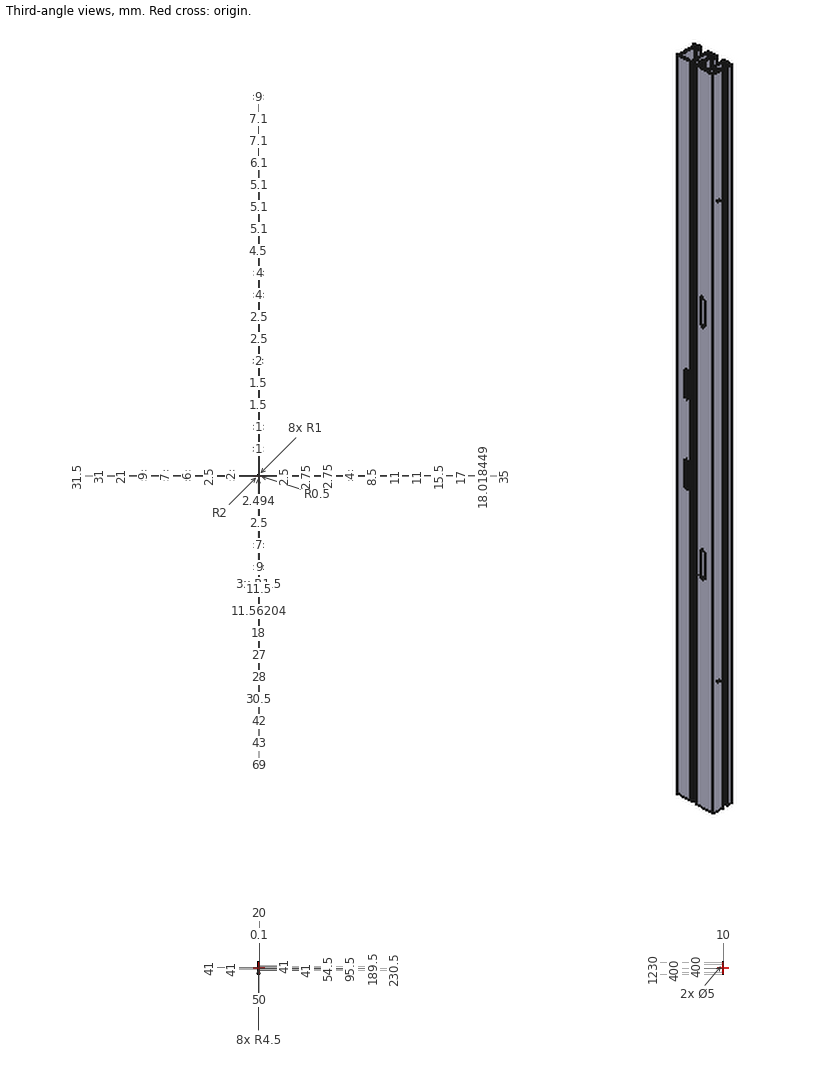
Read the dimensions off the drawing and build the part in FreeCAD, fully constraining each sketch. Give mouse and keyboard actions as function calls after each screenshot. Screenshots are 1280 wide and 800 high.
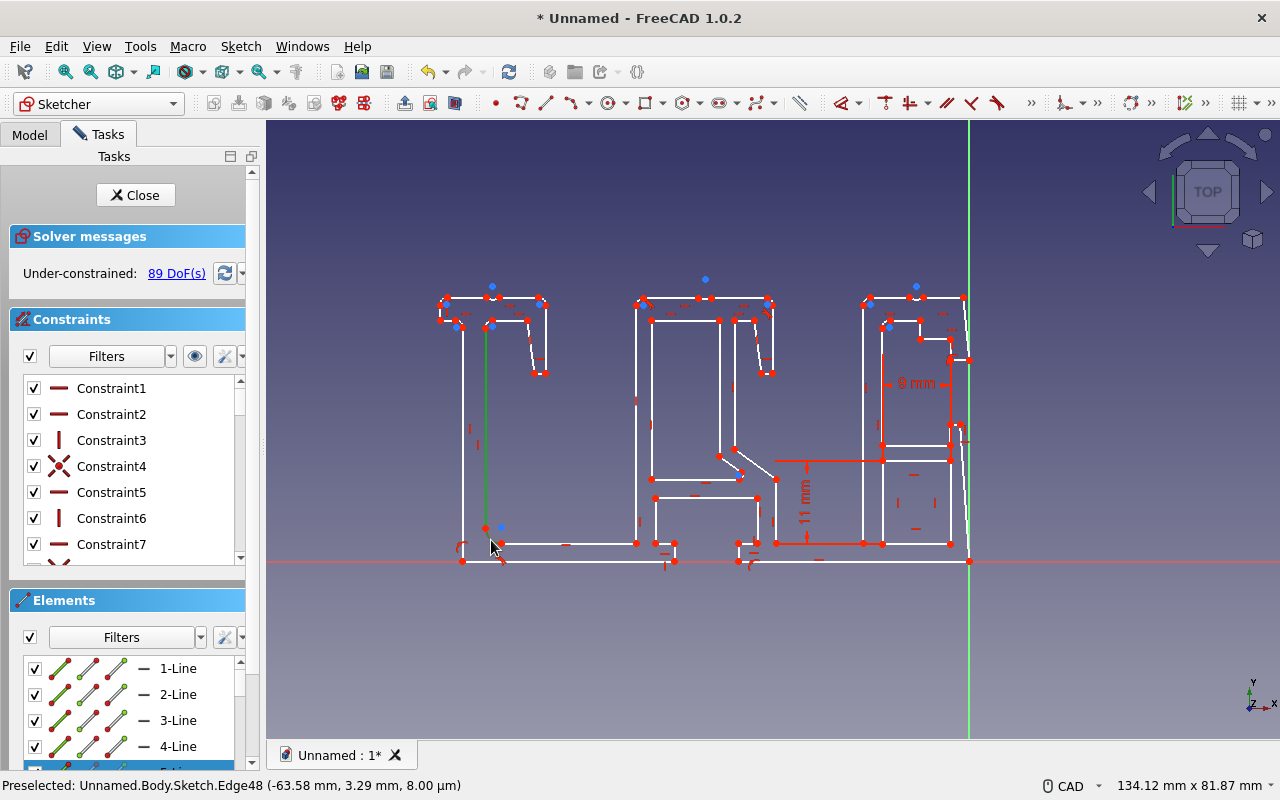
click(997, 104)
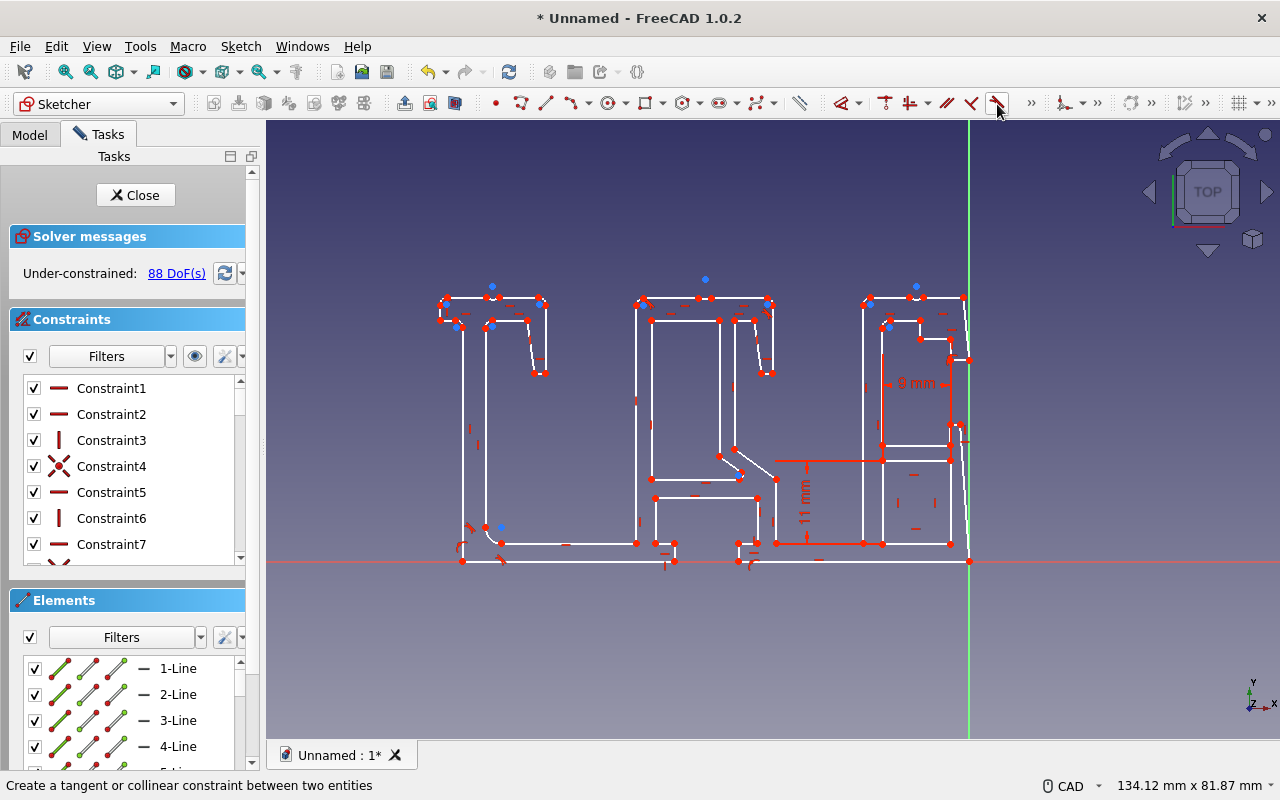
click(486, 468)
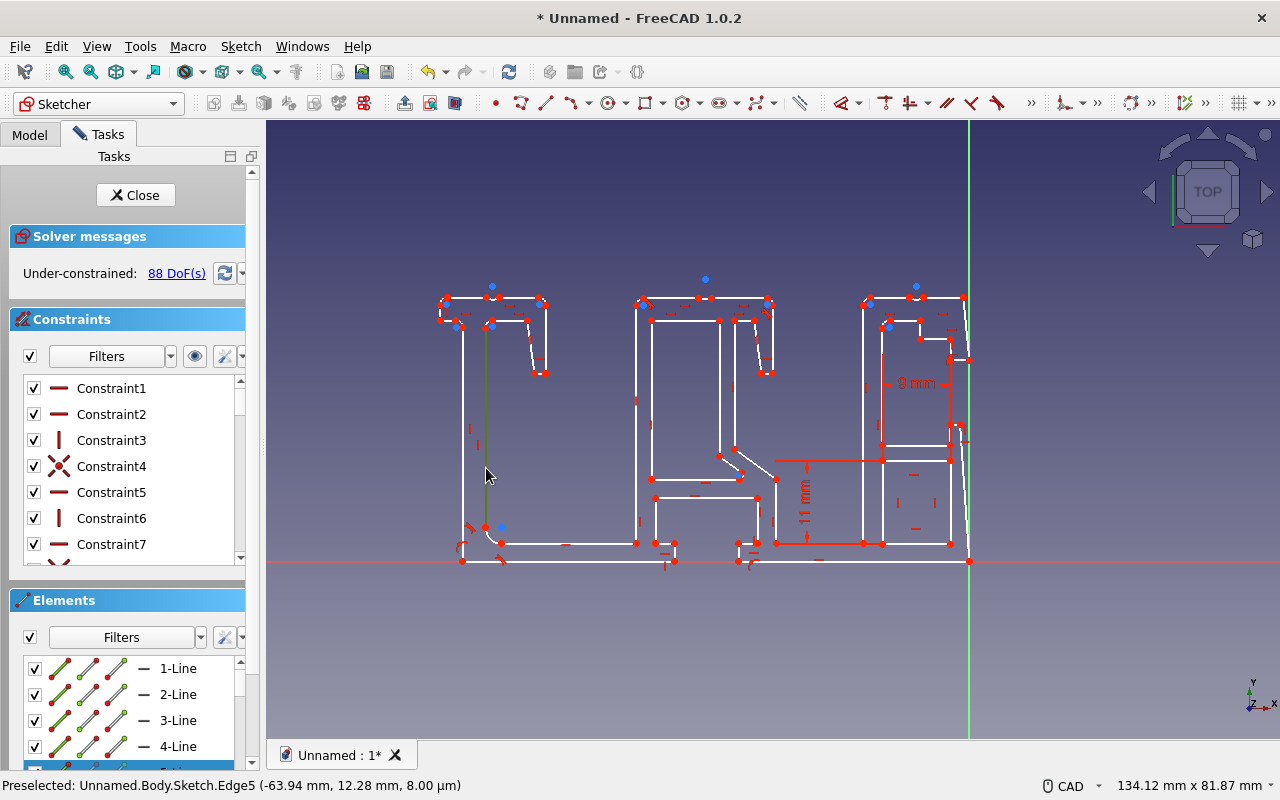
scroll(487, 323, up, 5)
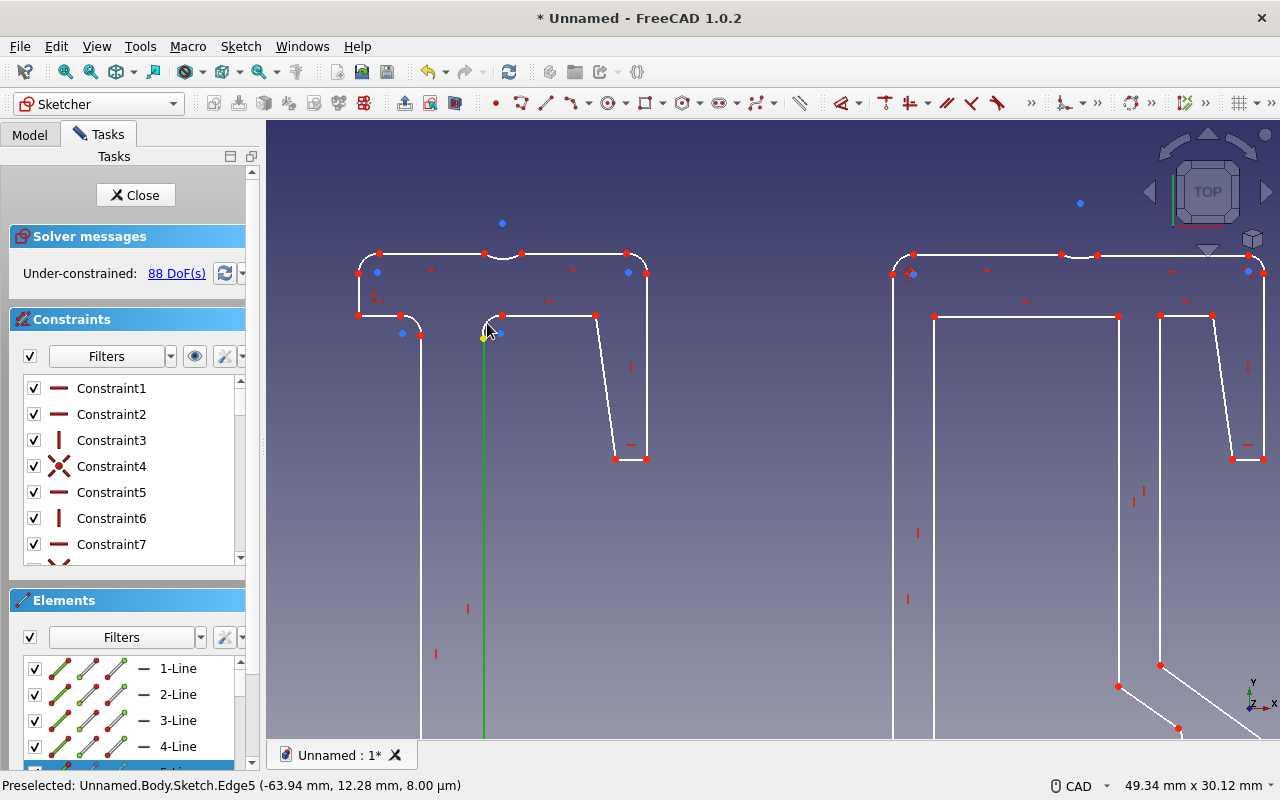
click(487, 322)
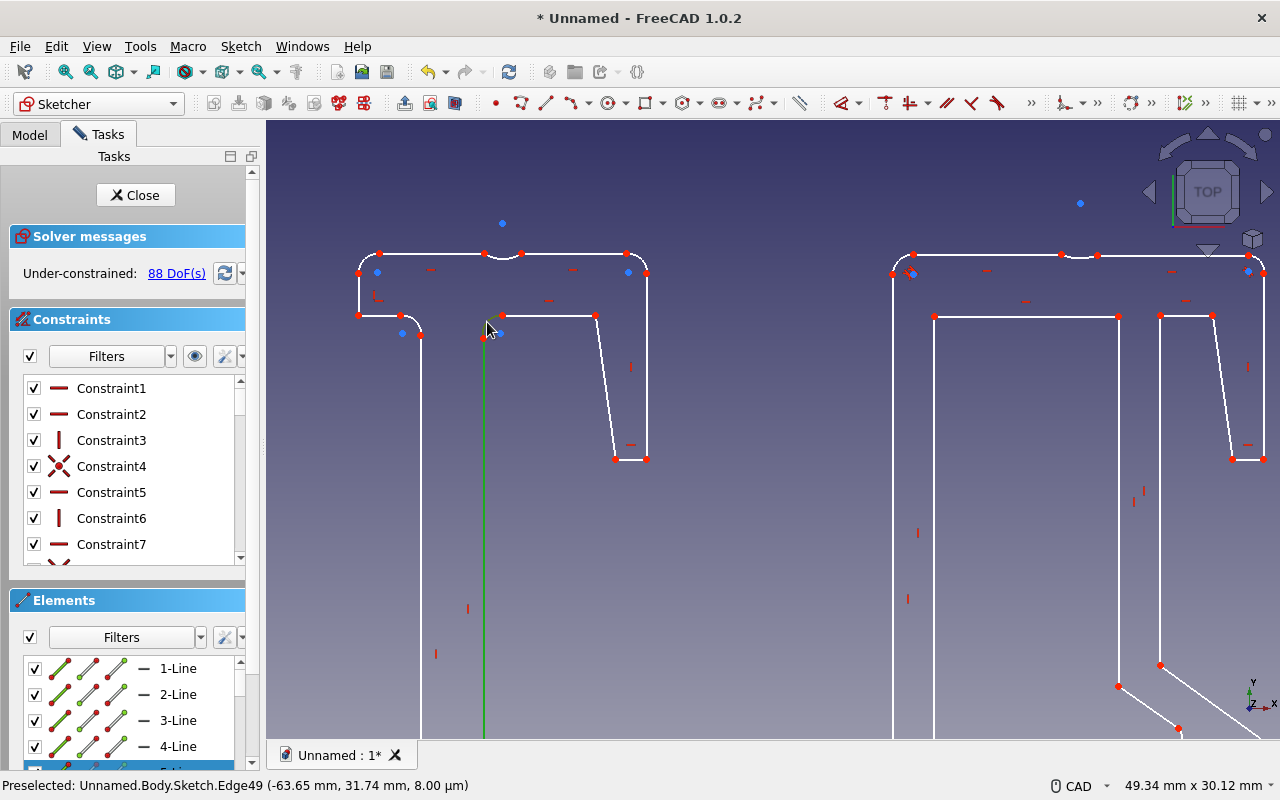
click(997, 104)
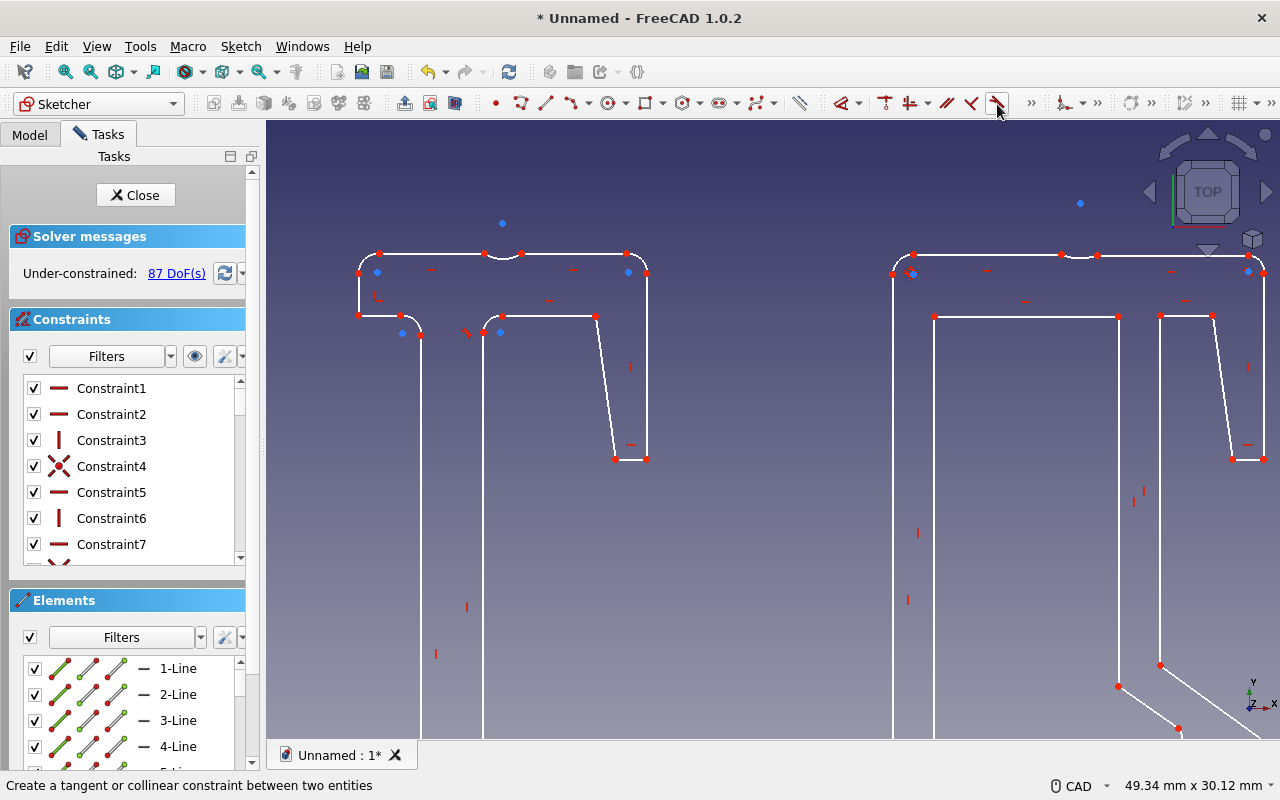
click(531, 316)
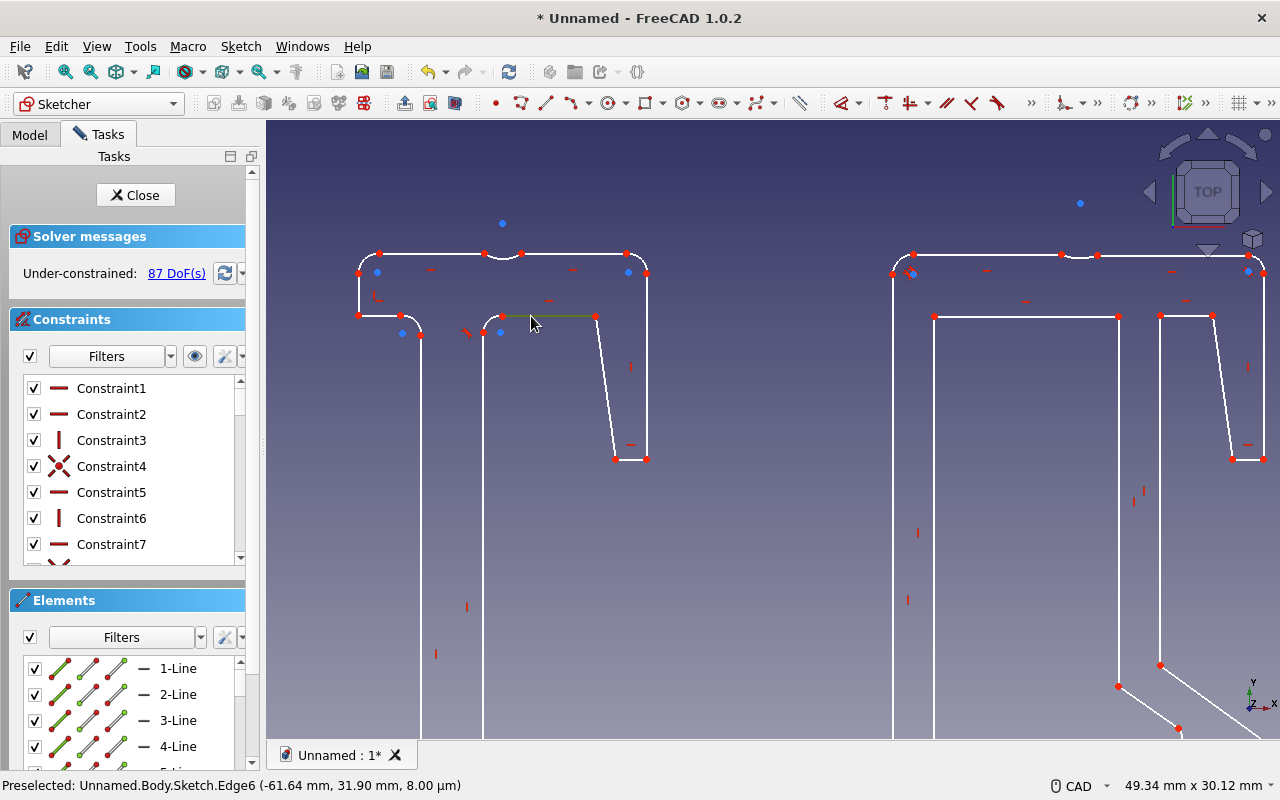
click(489, 320)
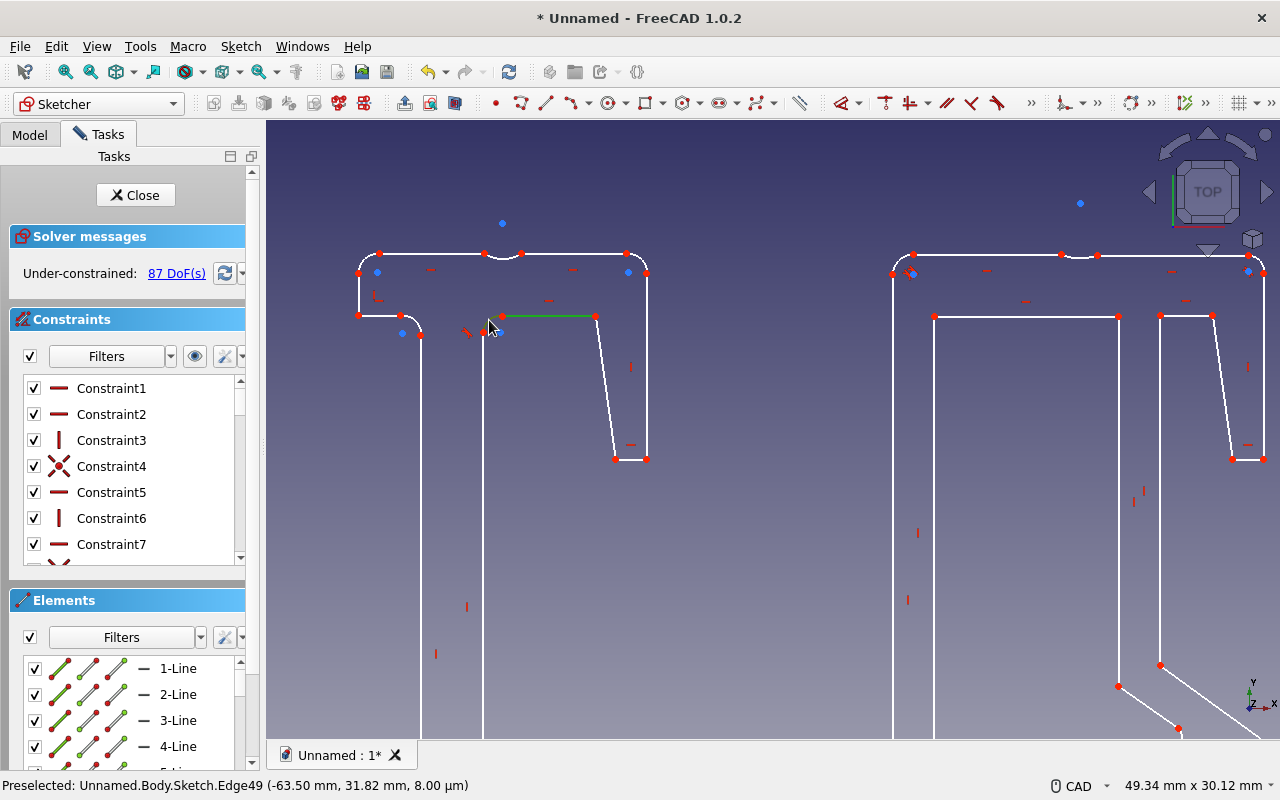
click(997, 104)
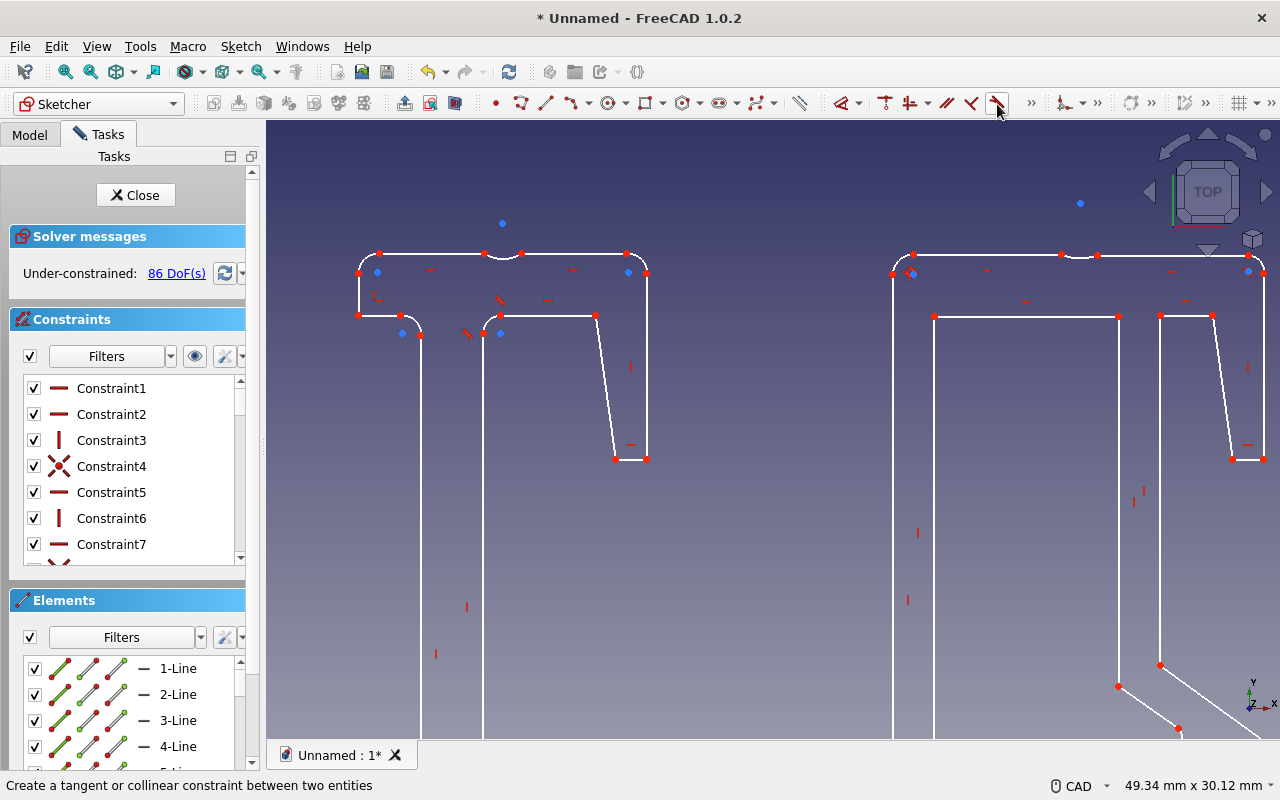
click(647, 404)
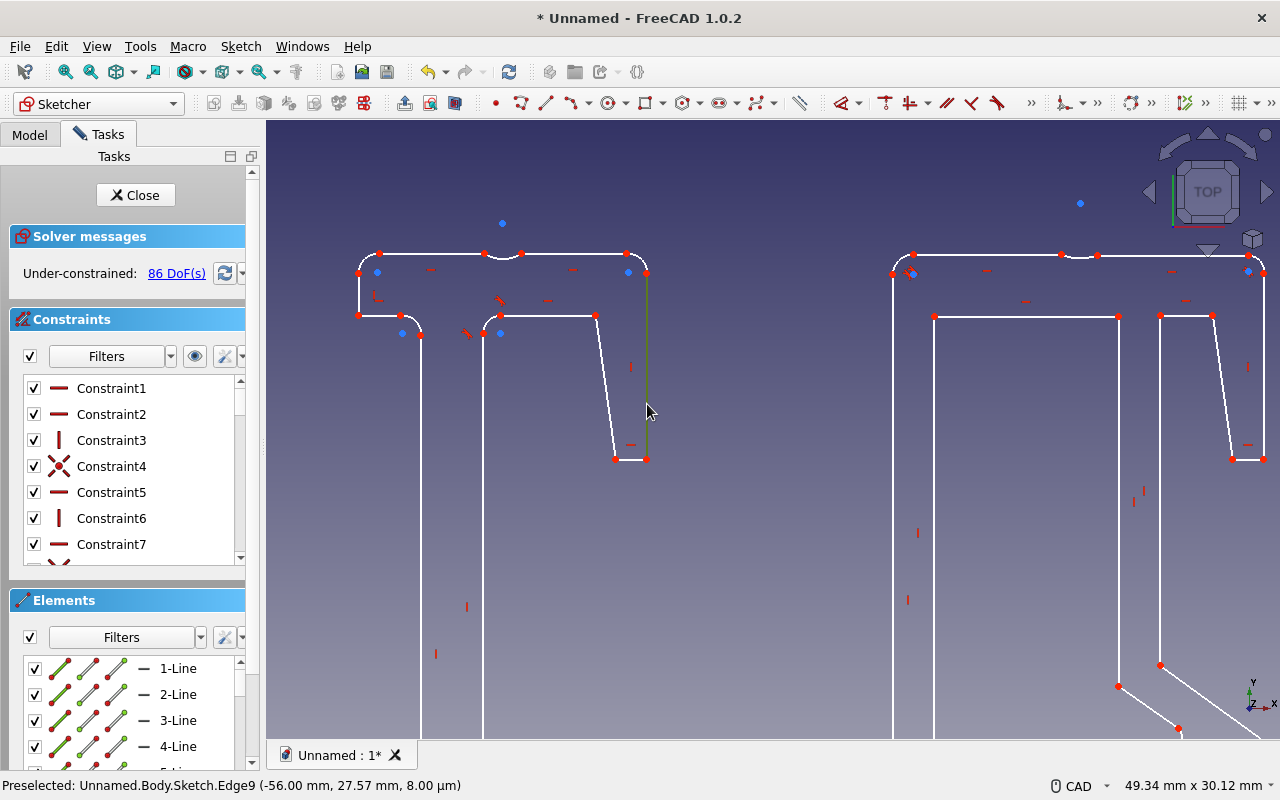
scroll(645, 265, up, 2)